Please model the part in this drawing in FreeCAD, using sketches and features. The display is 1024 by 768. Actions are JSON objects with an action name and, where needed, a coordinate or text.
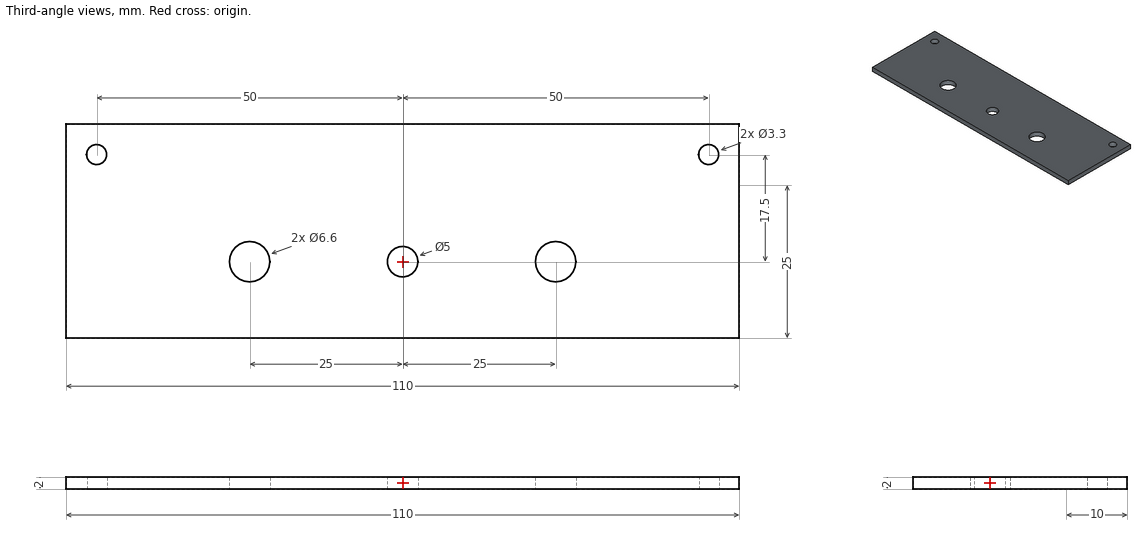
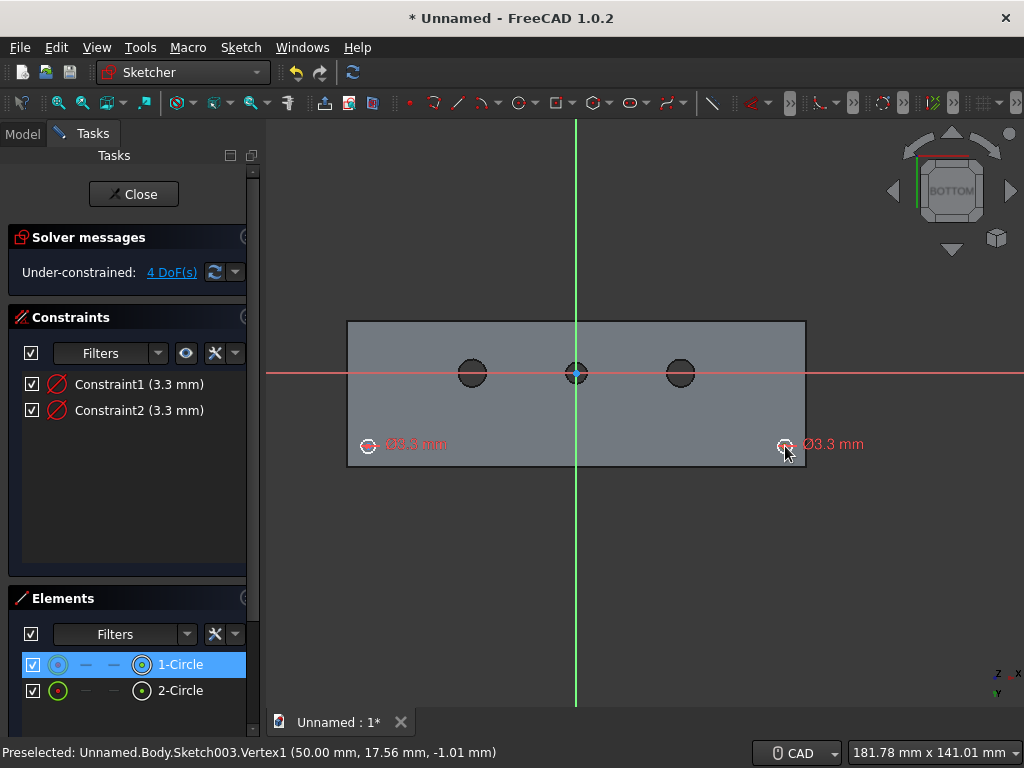
{"action": "left_click", "coordinate": [368, 446]}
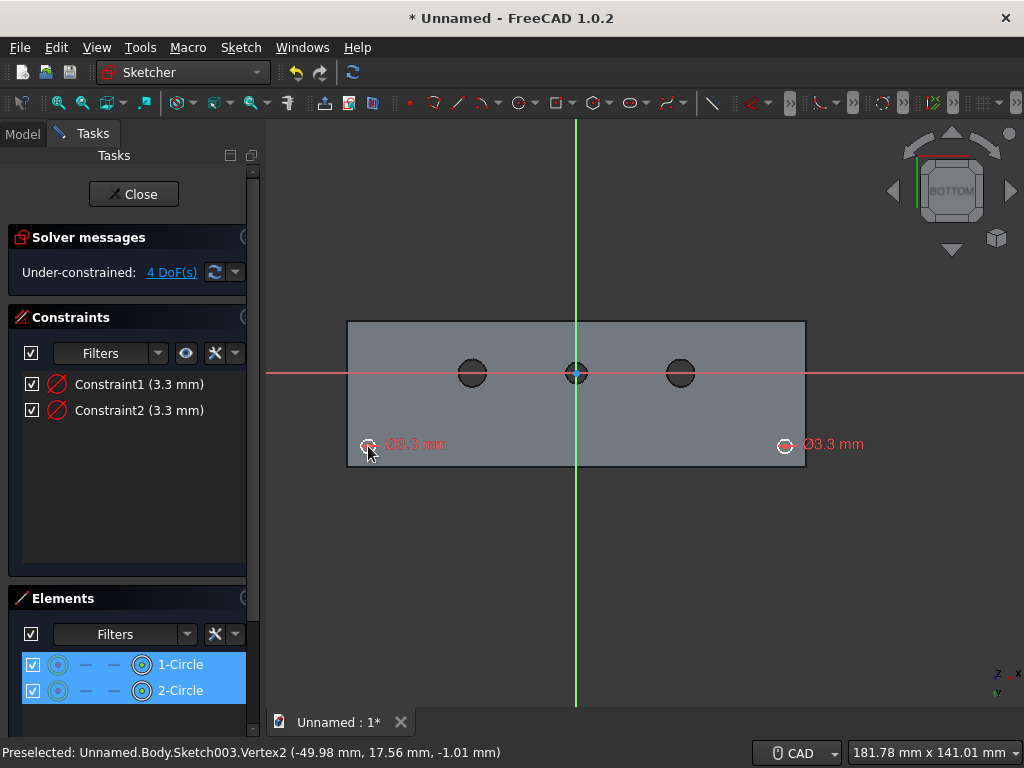
{"action": "key", "text": "h"}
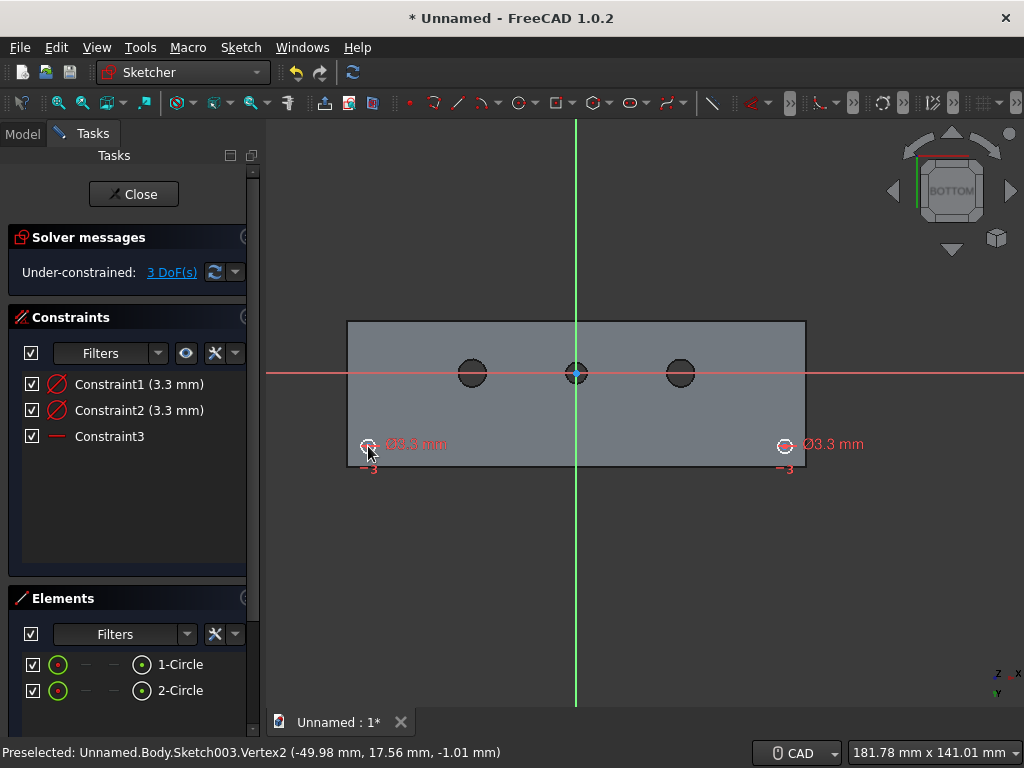
{"action": "left_click", "coordinate": [752, 104]}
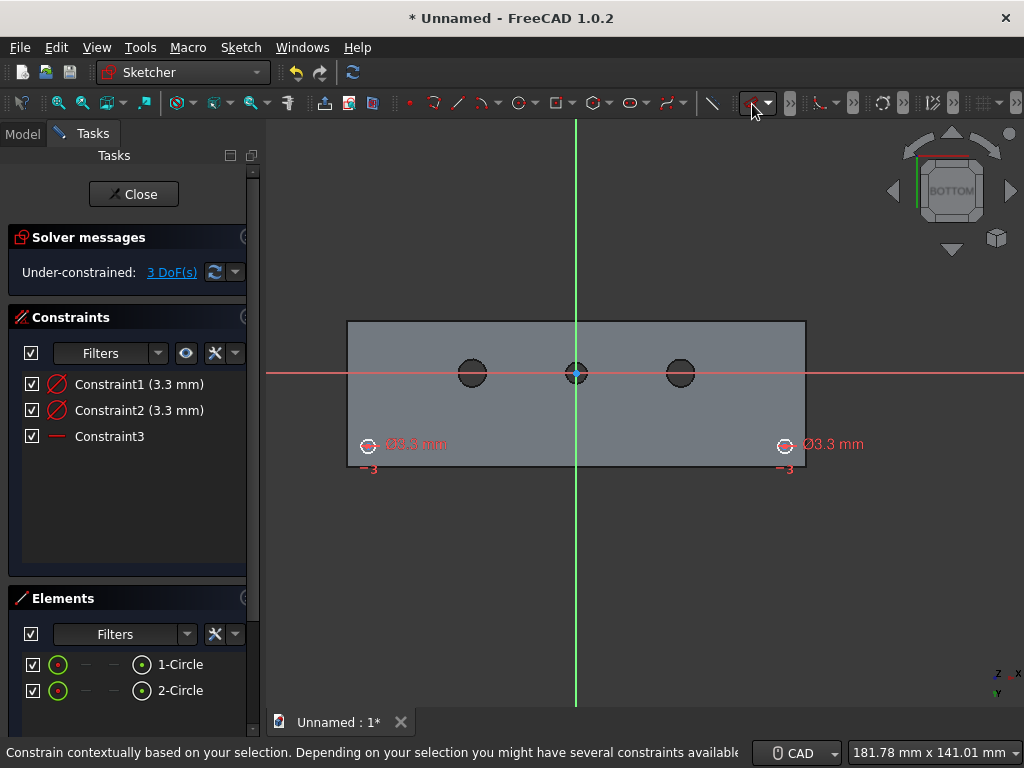
{"action": "left_click", "coordinate": [785, 446]}
{"action": "left_click", "coordinate": [681, 339]}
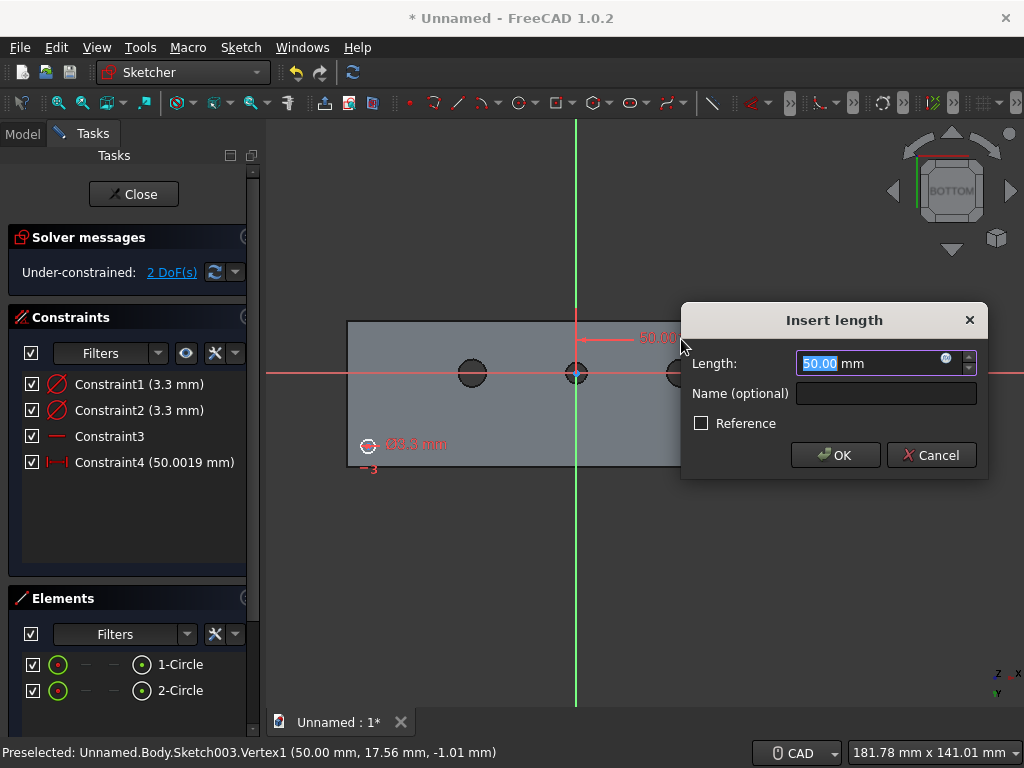
{"action": "type", "text": "50"}
{"action": "key", "text": "Return"}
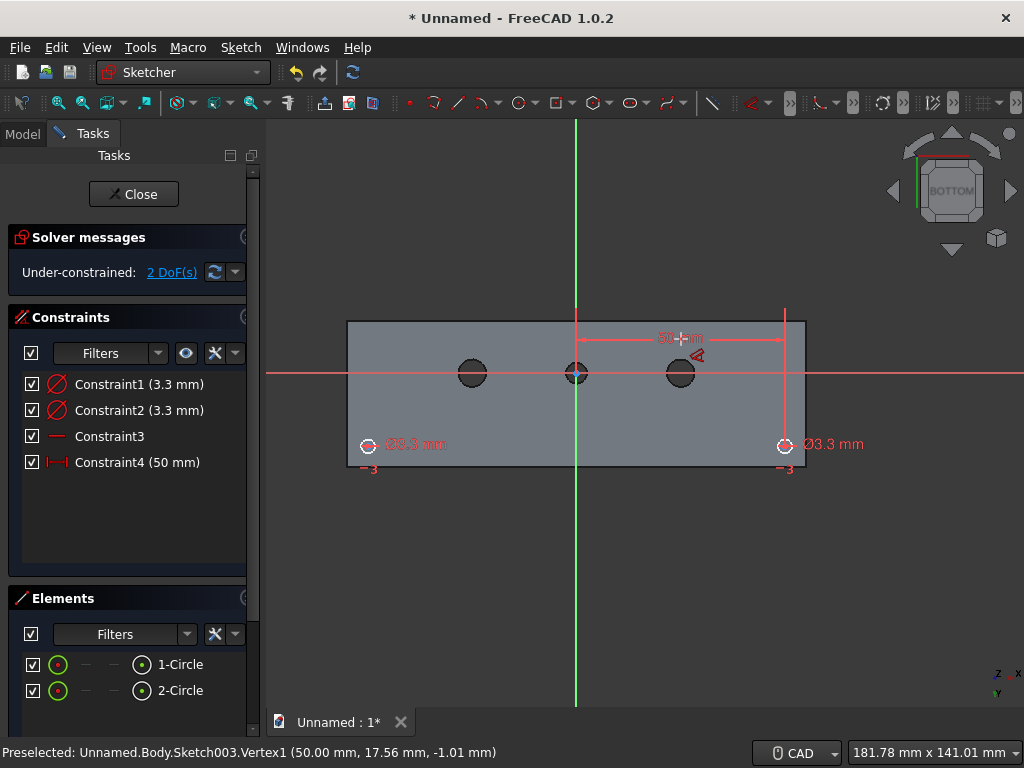
{"action": "left_click", "coordinate": [368, 446]}
{"action": "left_click", "coordinate": [472, 339]}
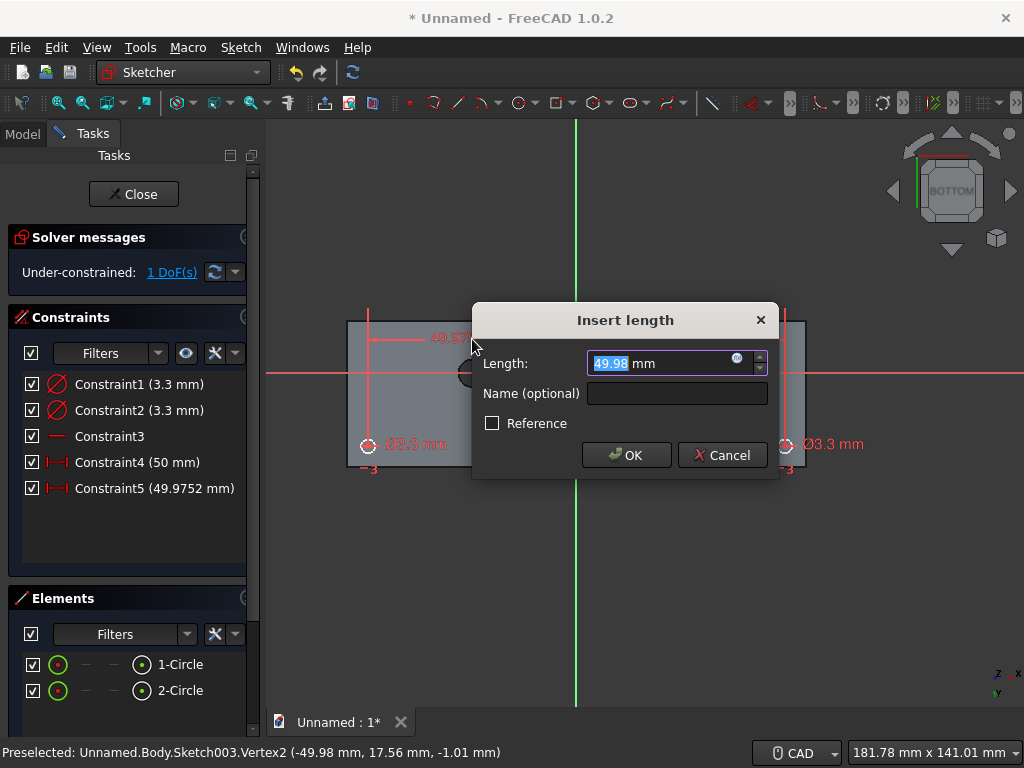
{"action": "type", "text": "50"}
{"action": "key", "text": "Return"}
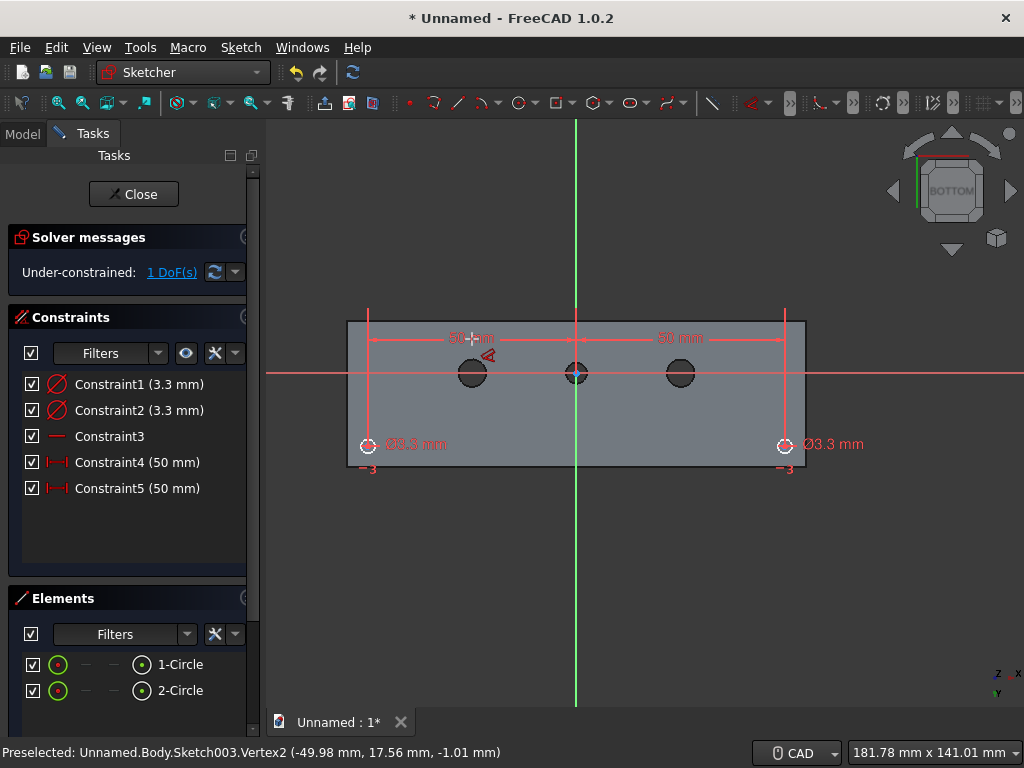
{"action": "left_click", "coordinate": [785, 446]}
{"action": "left_click", "coordinate": [819, 410]}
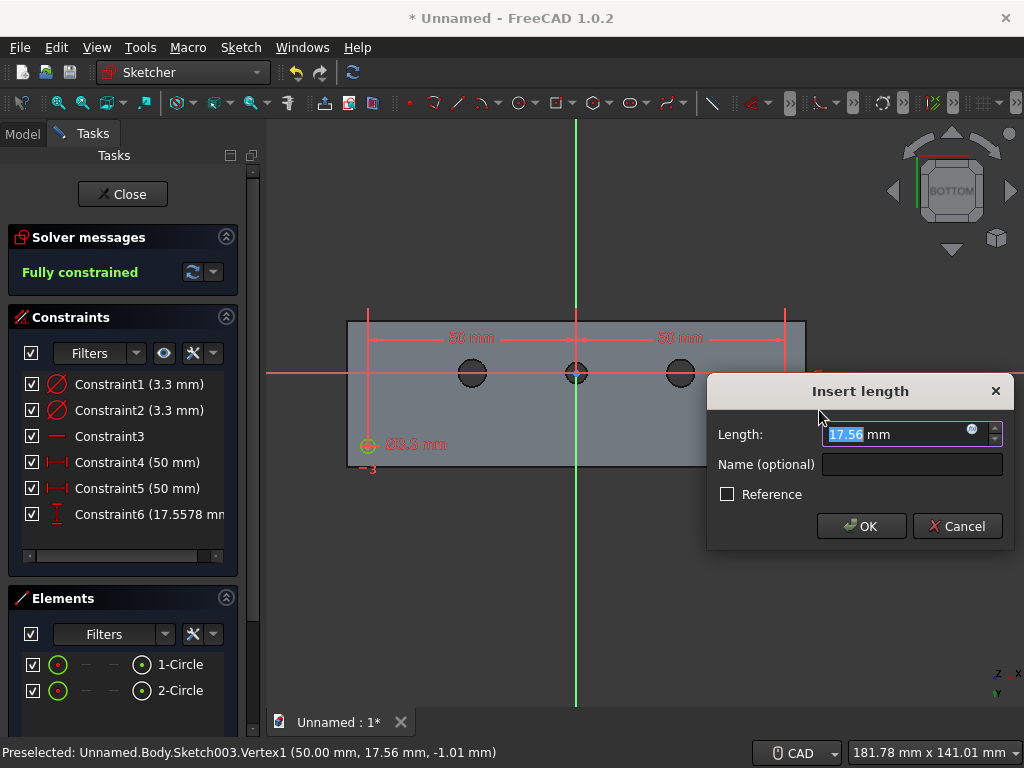
{"action": "type", "text": "17.5"}
{"action": "key", "text": "Return"}
{"action": "key", "text": "Escape"}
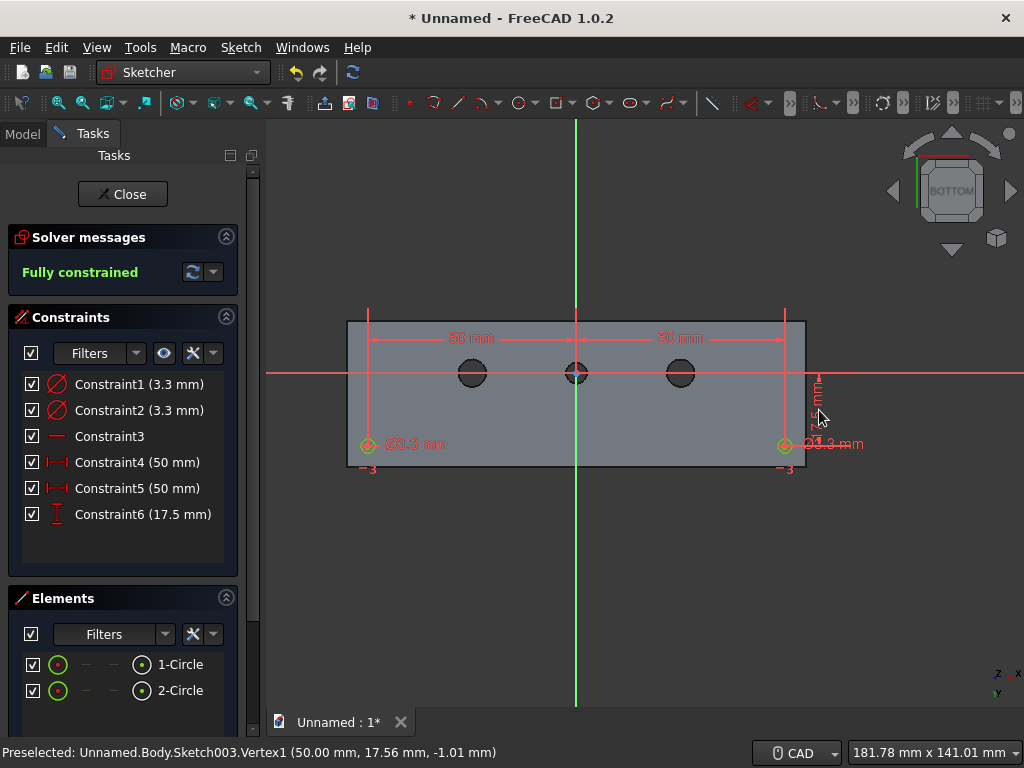
{"action": "left_click", "coordinate": [123, 194]}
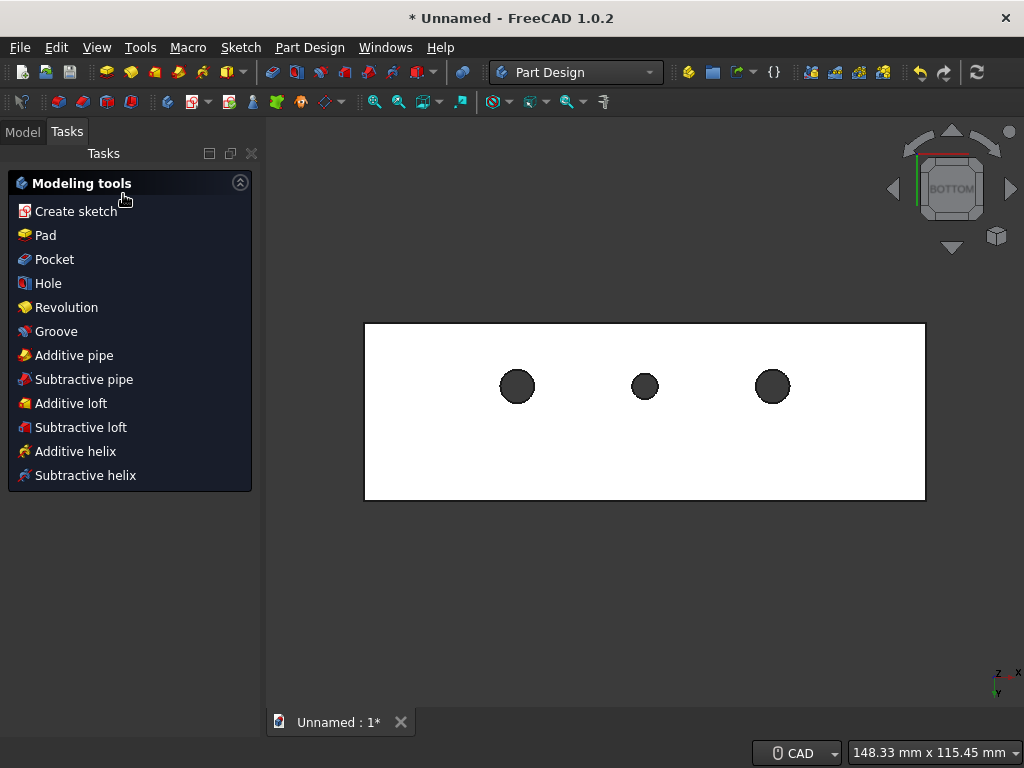
{"action": "left_click", "coordinate": [274, 72]}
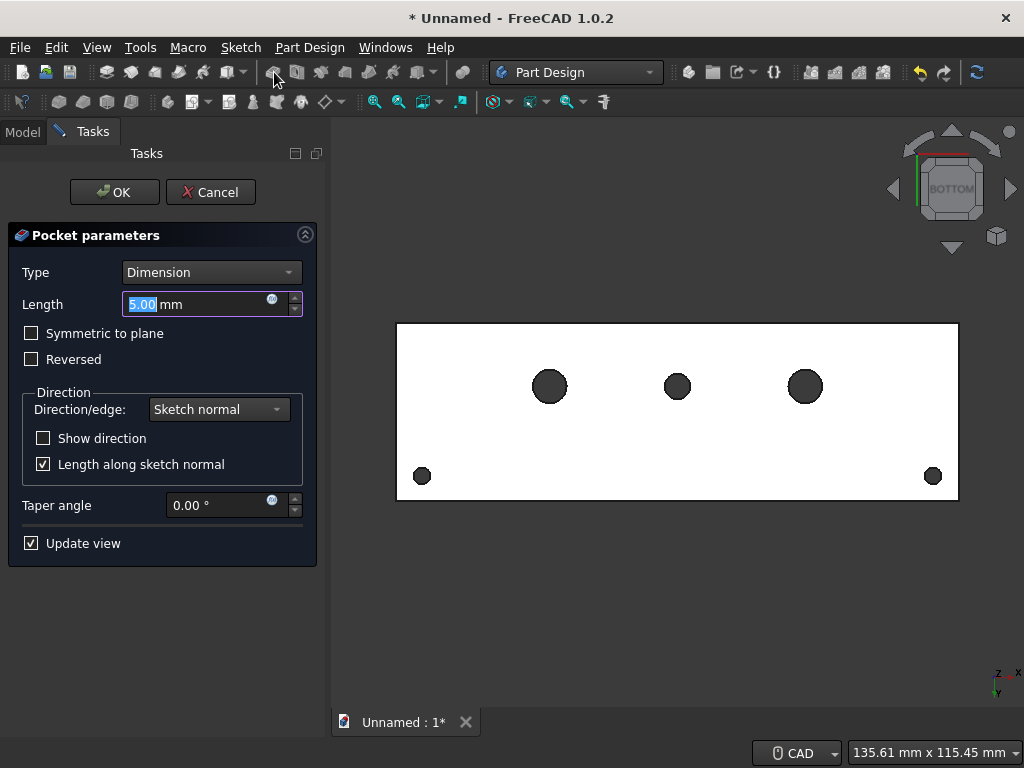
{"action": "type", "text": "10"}
{"action": "key", "text": "Tab"}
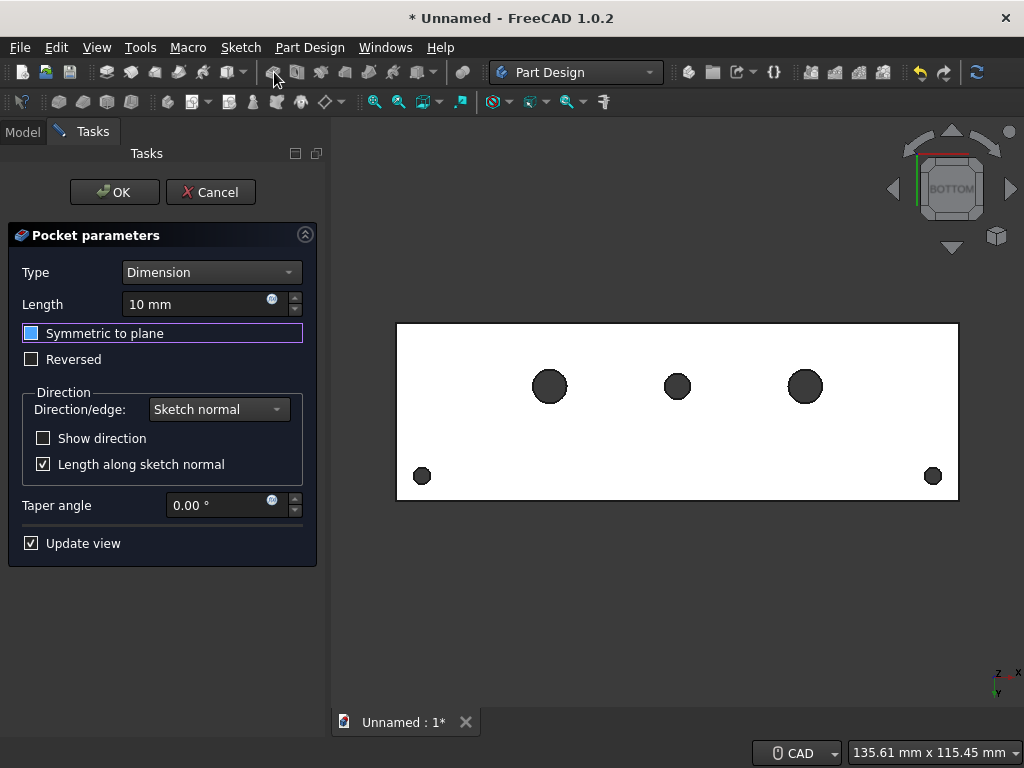
{"action": "left_click", "coordinate": [115, 192]}